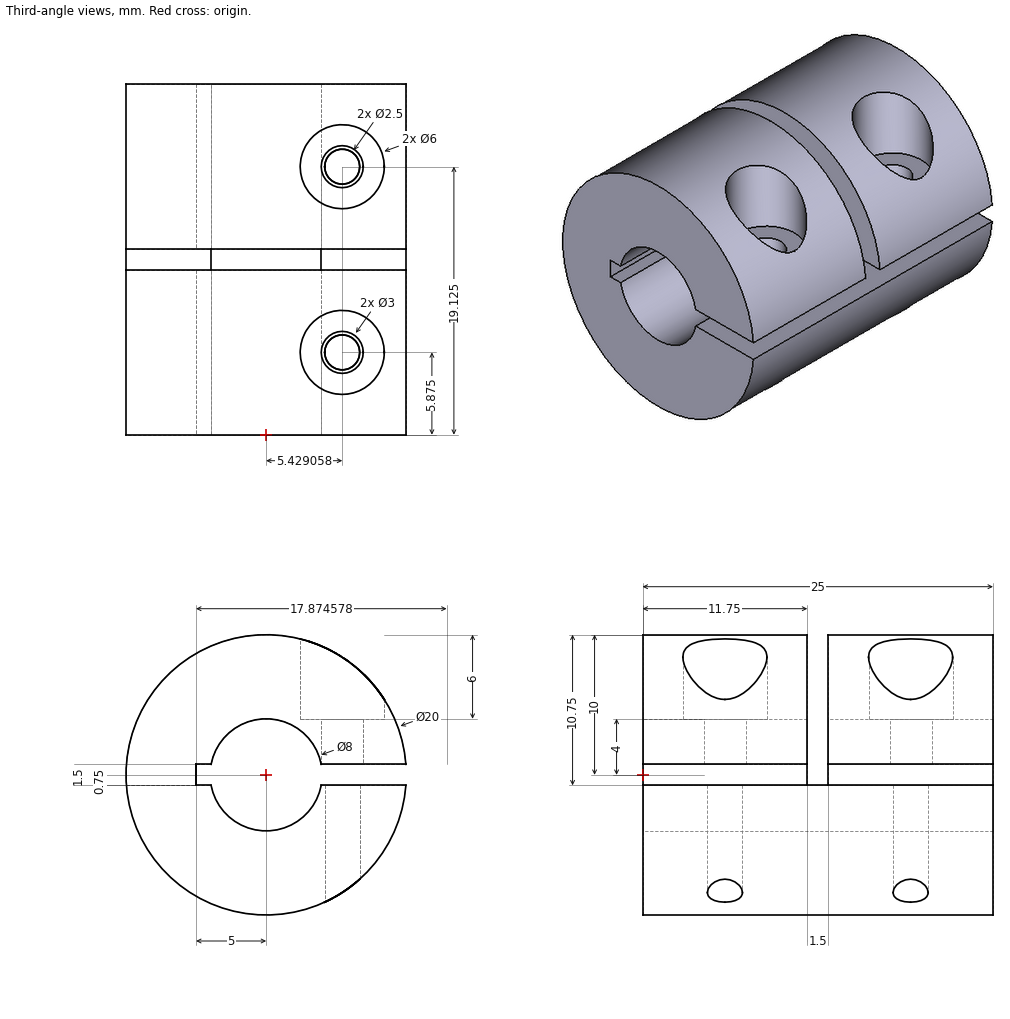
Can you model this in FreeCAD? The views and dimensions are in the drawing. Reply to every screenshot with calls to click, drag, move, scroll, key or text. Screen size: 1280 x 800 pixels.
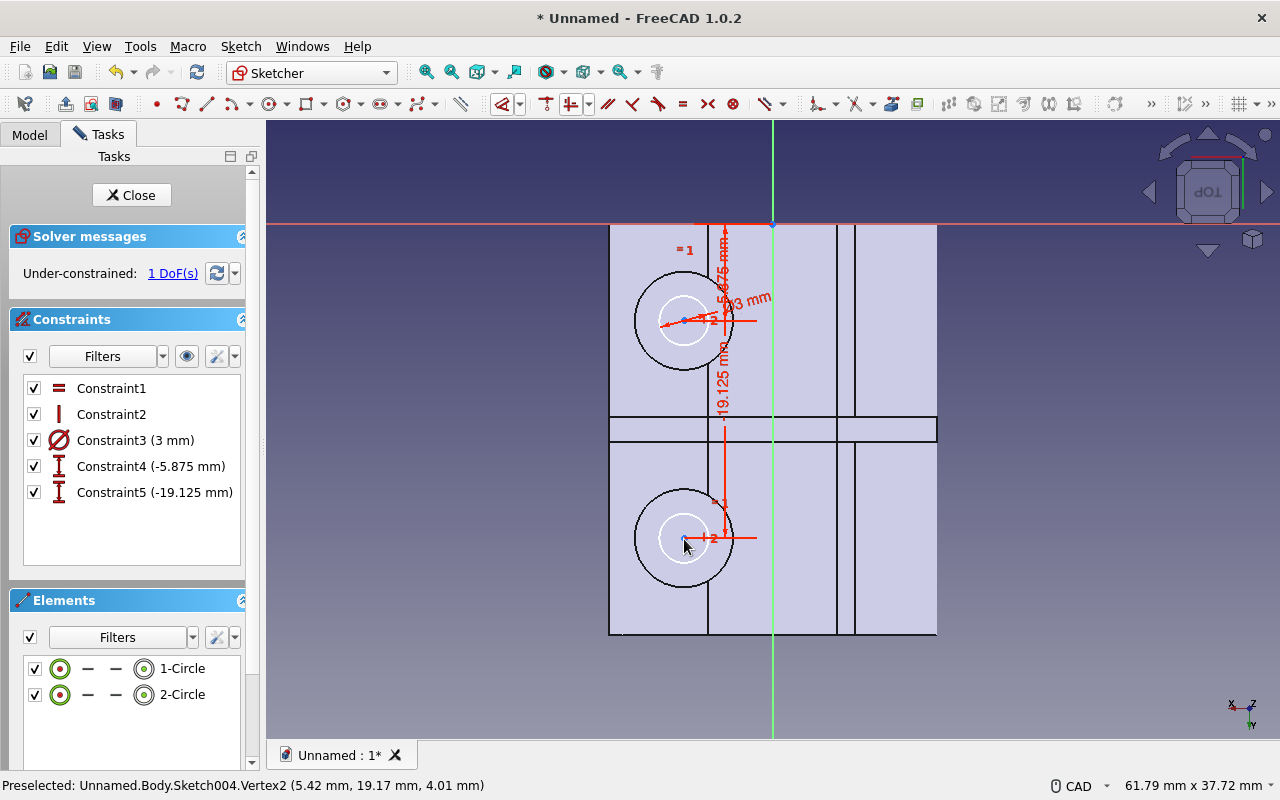
click(684, 321)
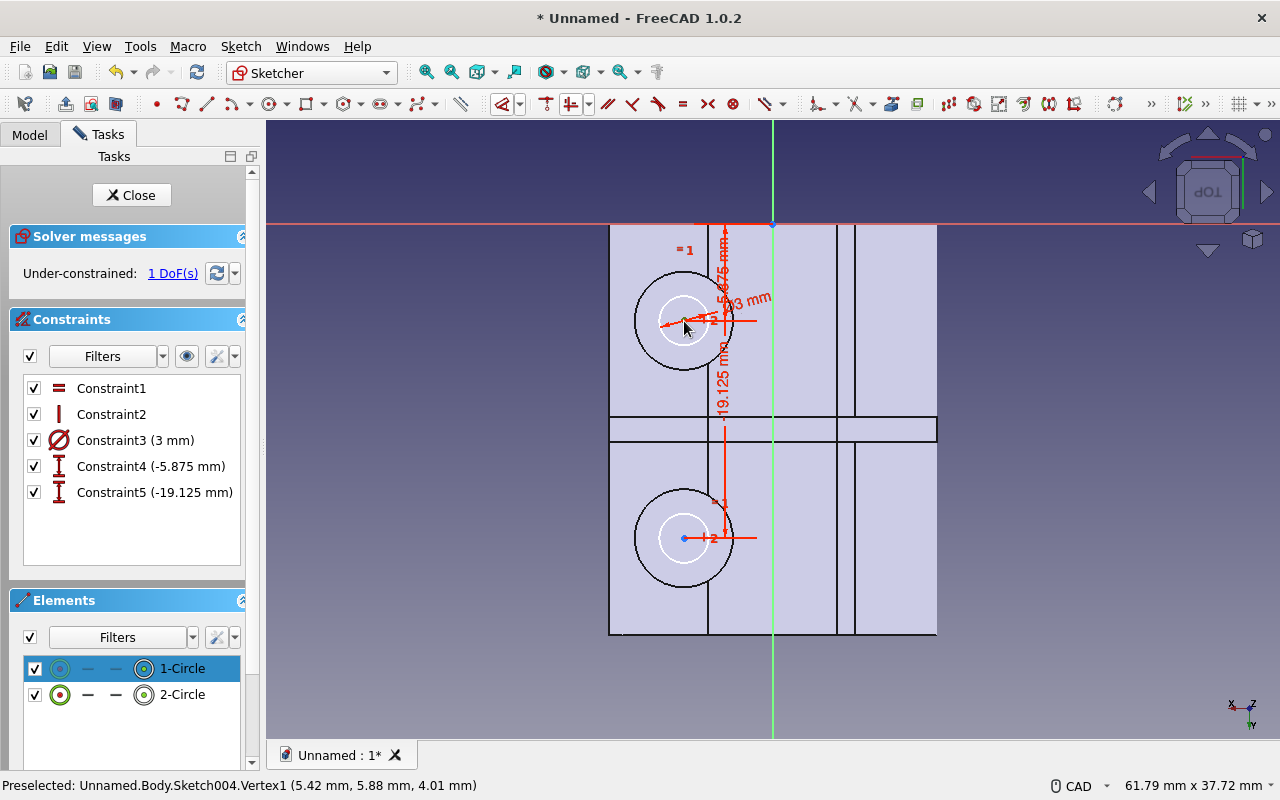
click(520, 104)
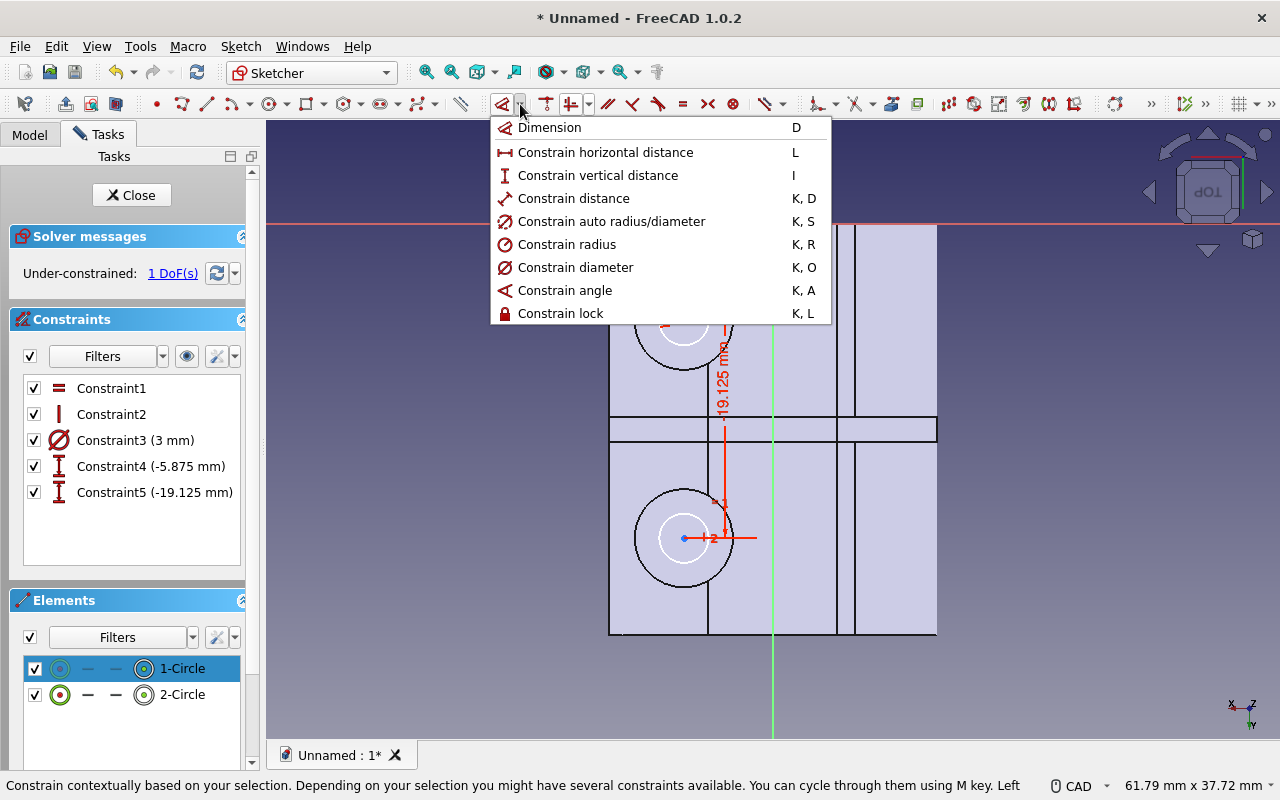
click(661, 152)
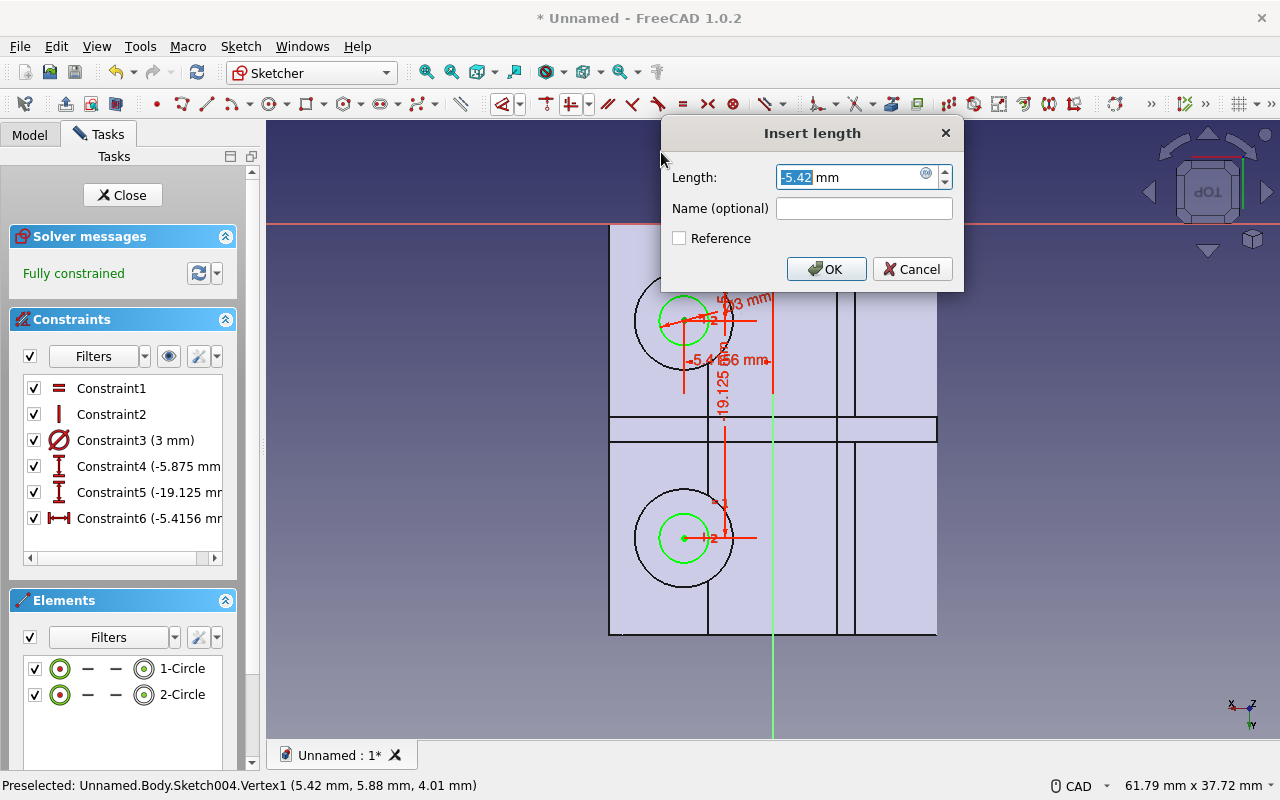
text(-5.429058)
key(Return)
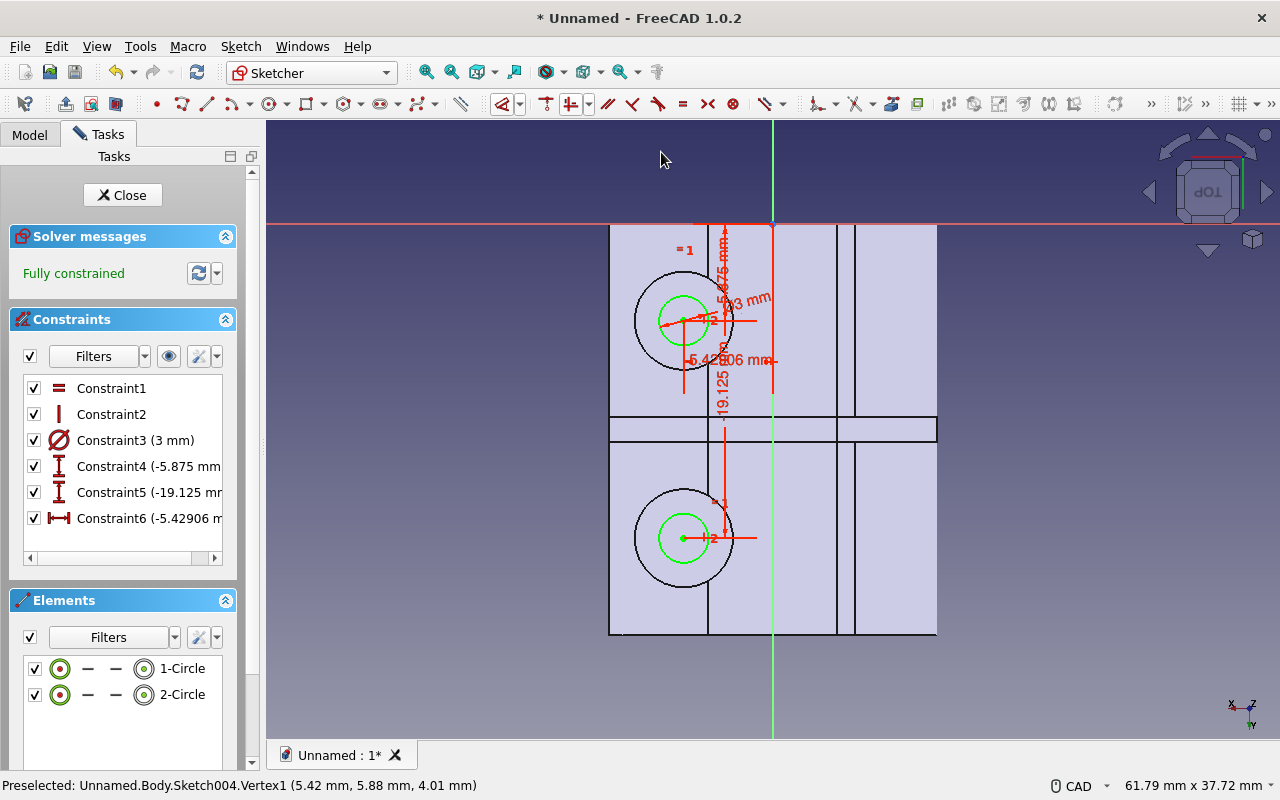
click(123, 195)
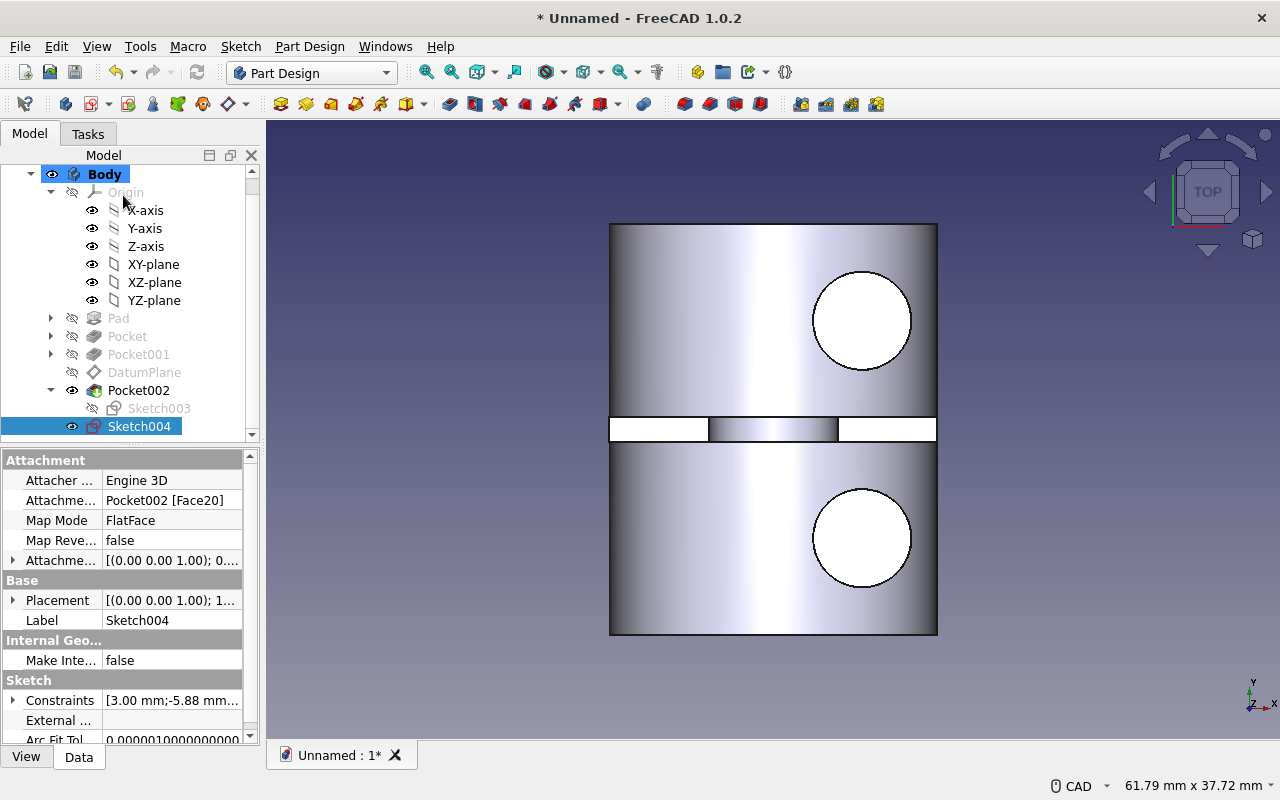
click(450, 104)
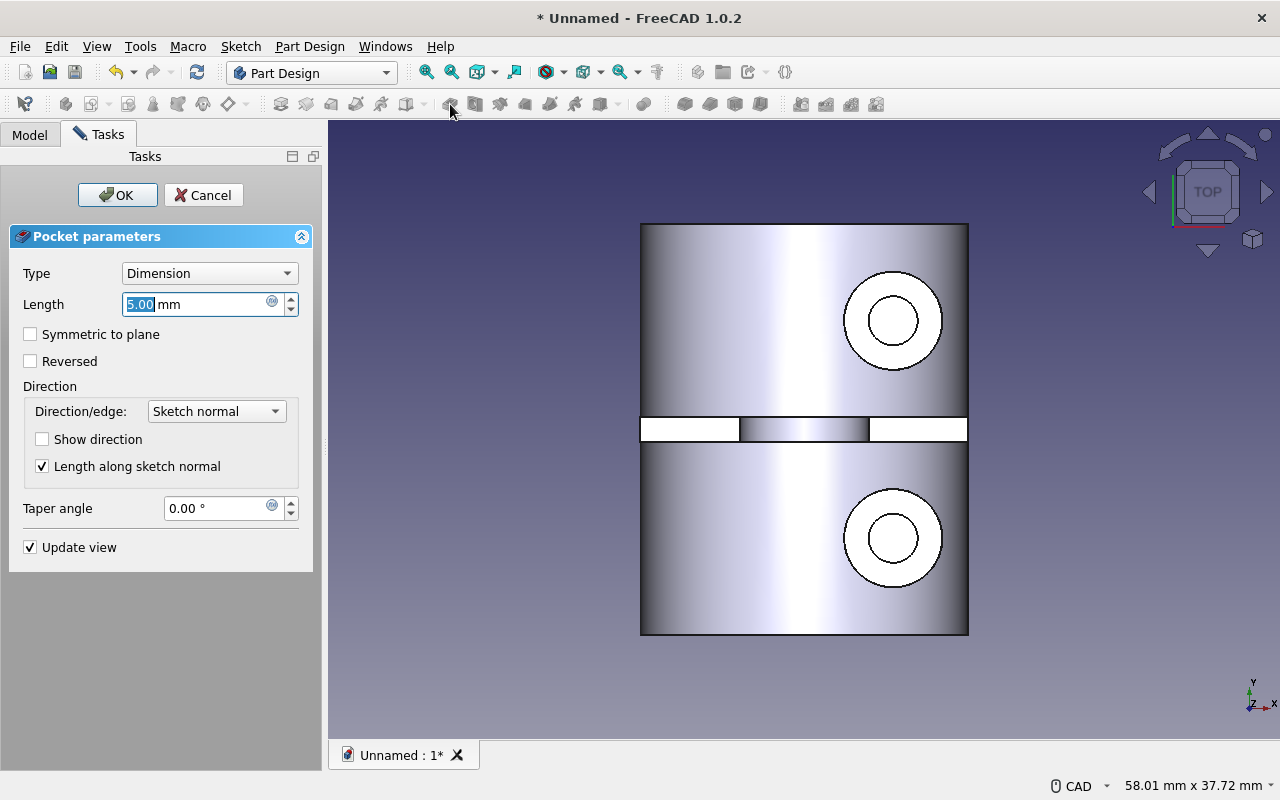
text(4)
key(Tab)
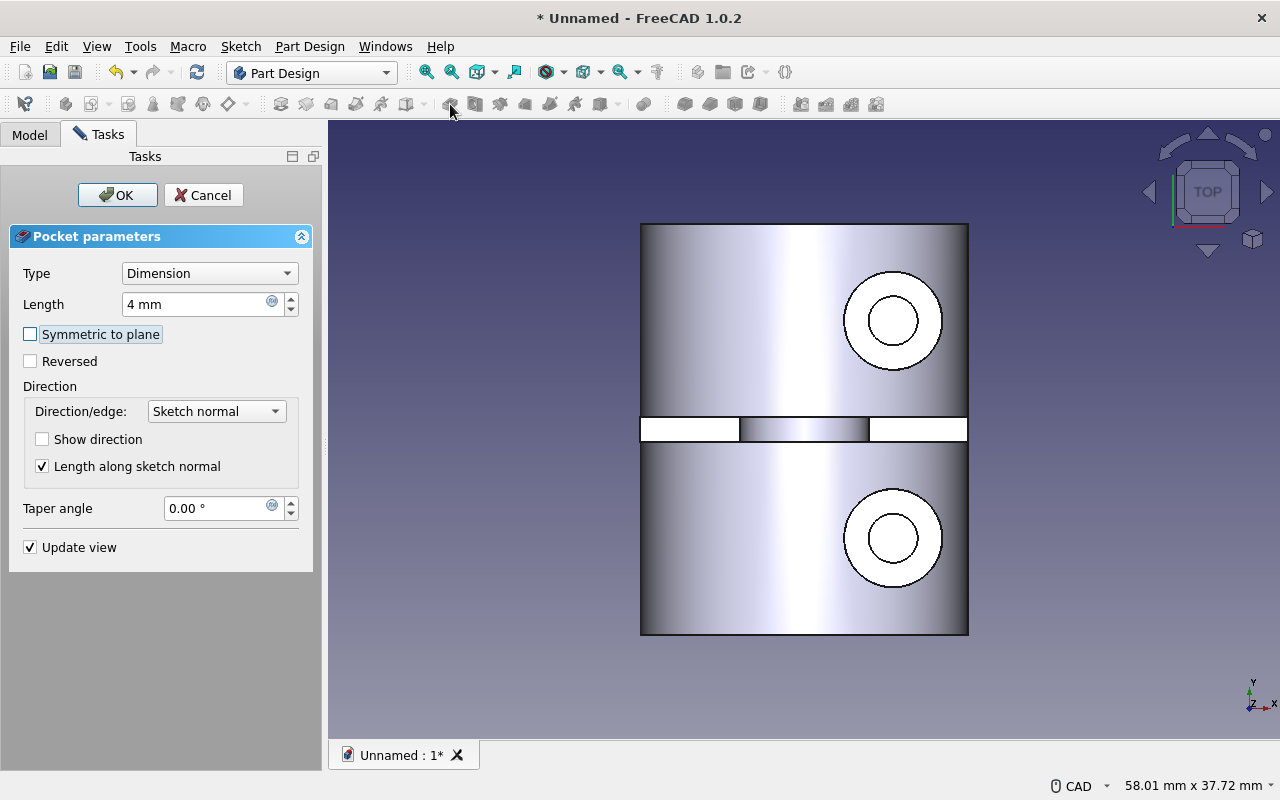
click(118, 195)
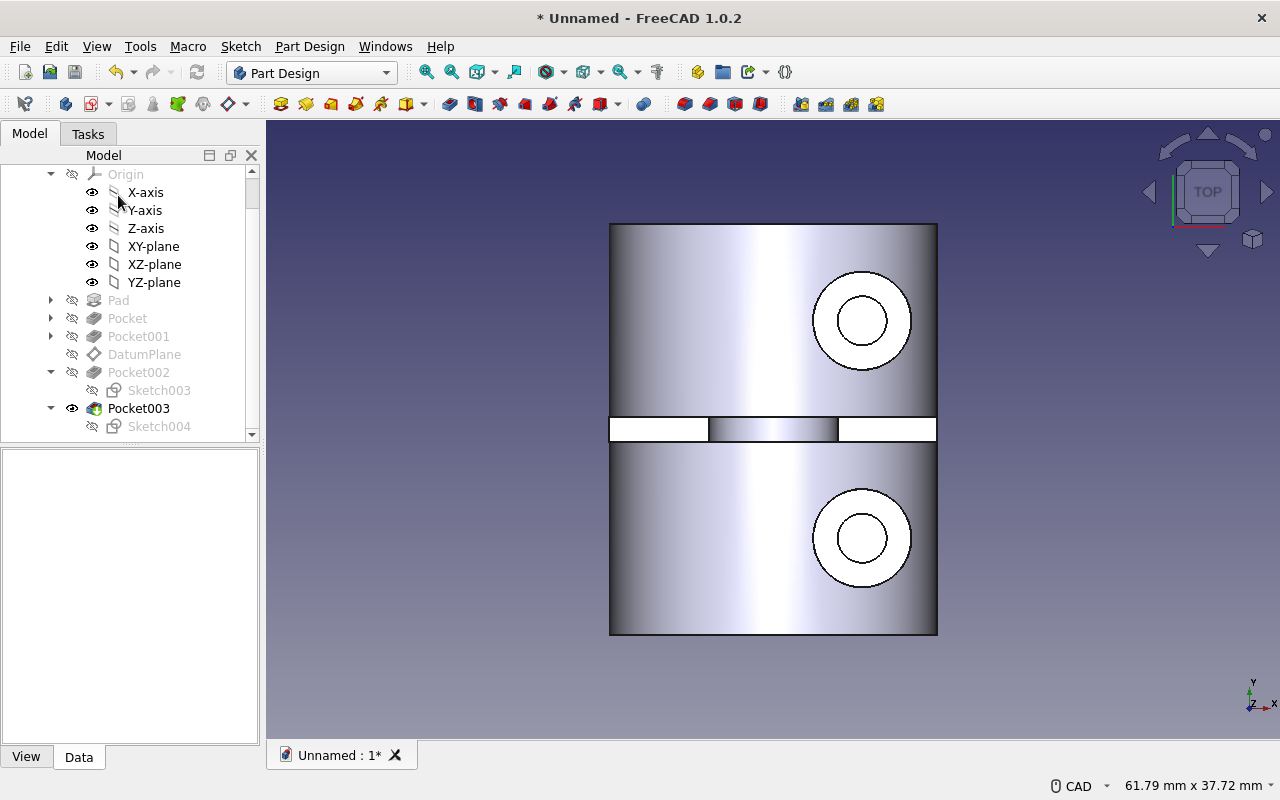
click(887, 429)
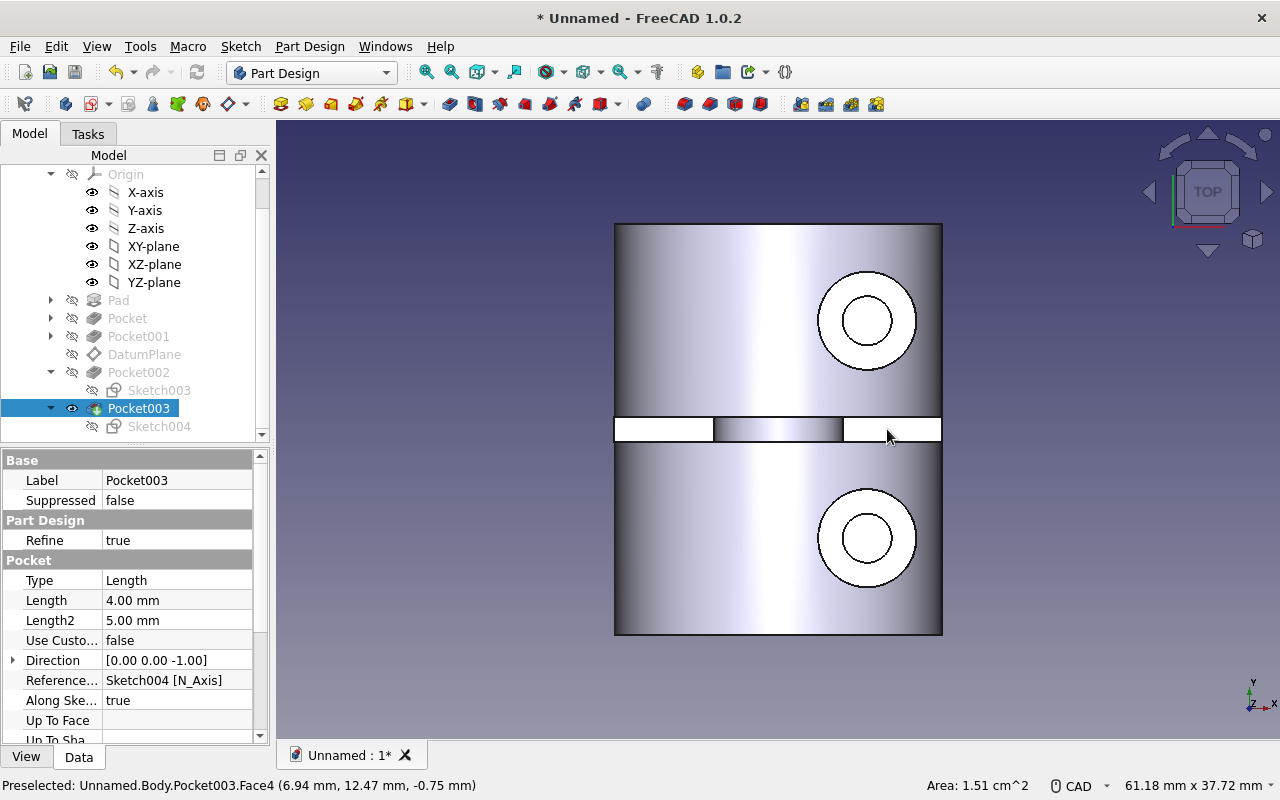
click(90, 104)